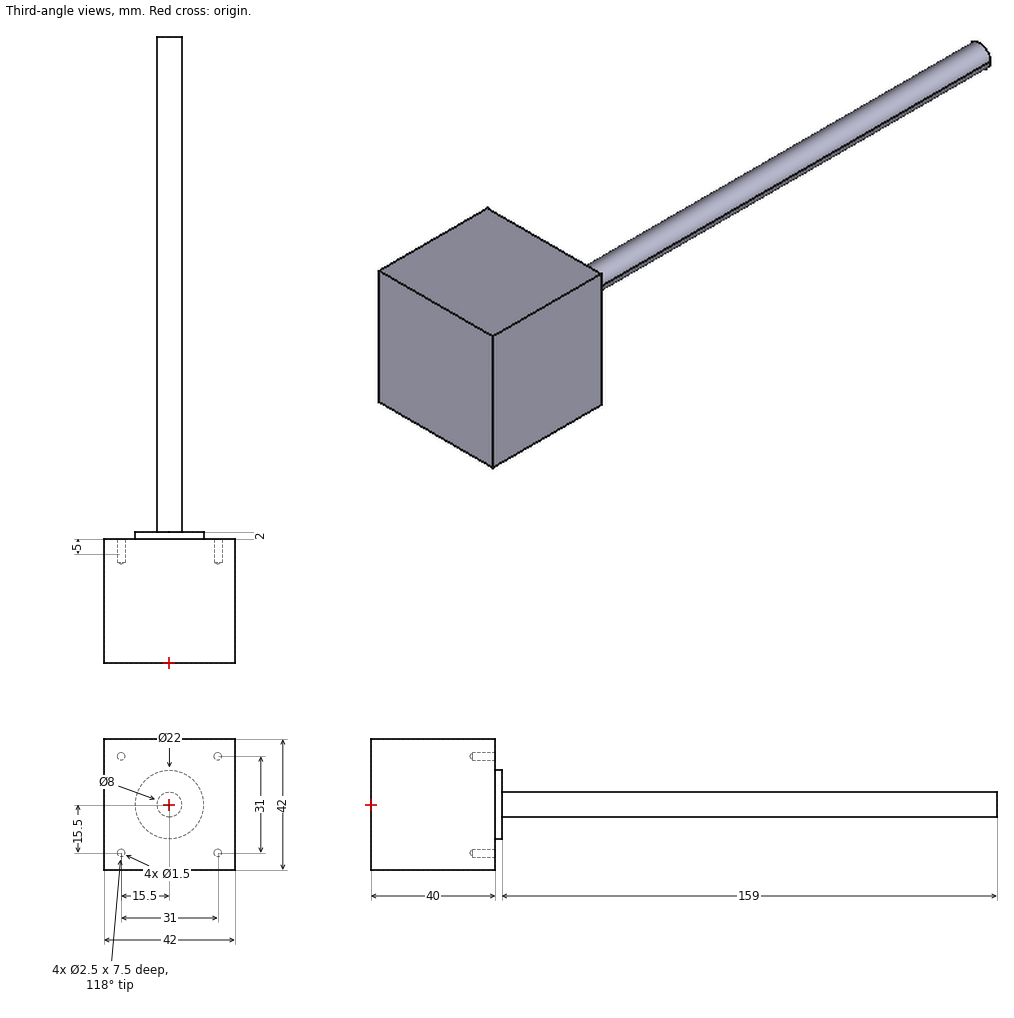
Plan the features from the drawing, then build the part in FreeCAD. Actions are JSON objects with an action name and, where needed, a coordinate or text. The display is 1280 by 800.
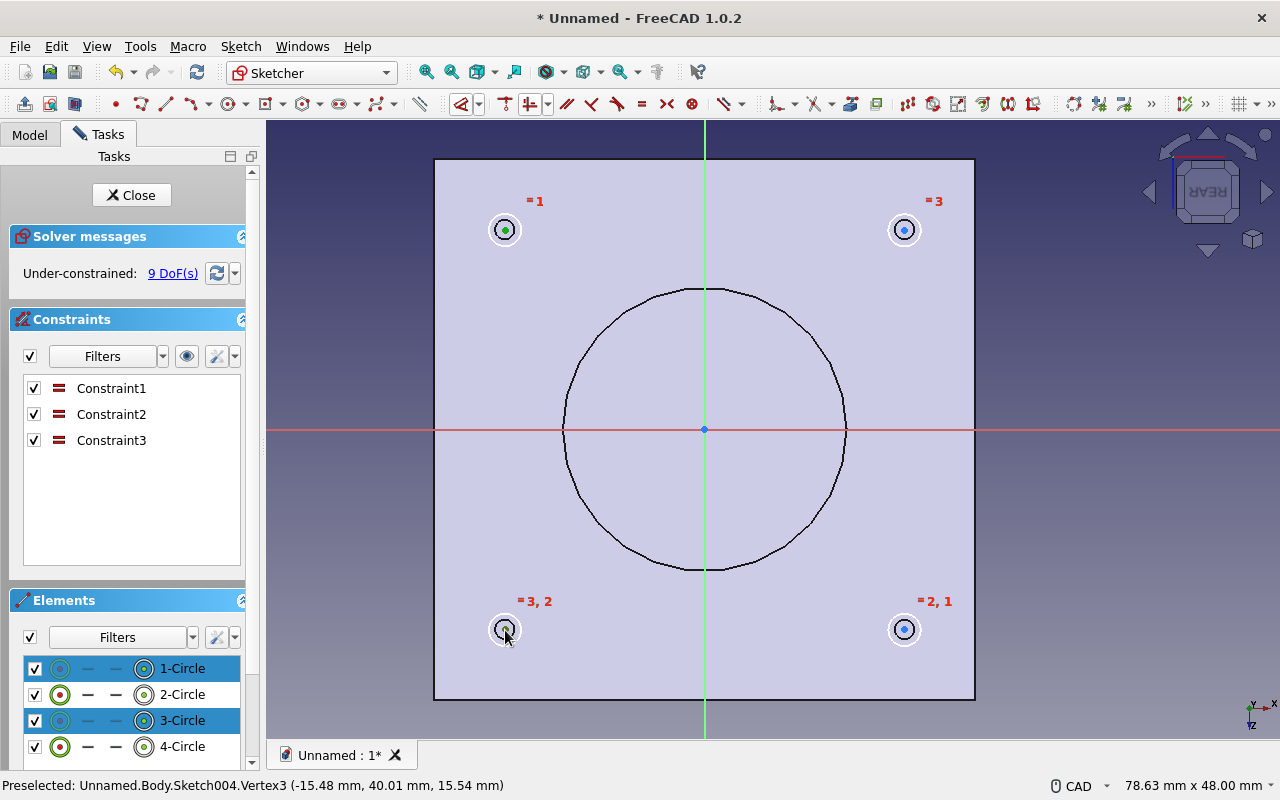
{"action": "key", "text": "v"}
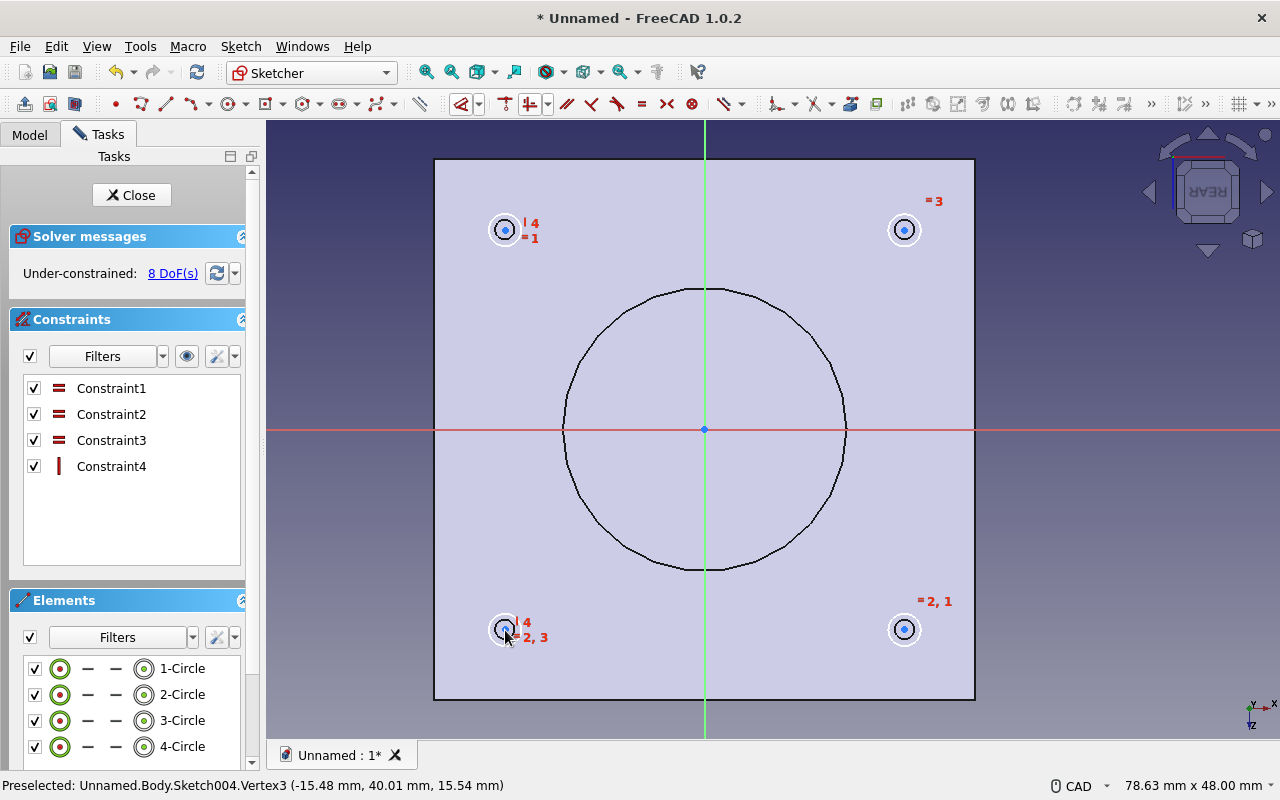
{"action": "left_click", "coordinate": [905, 630]}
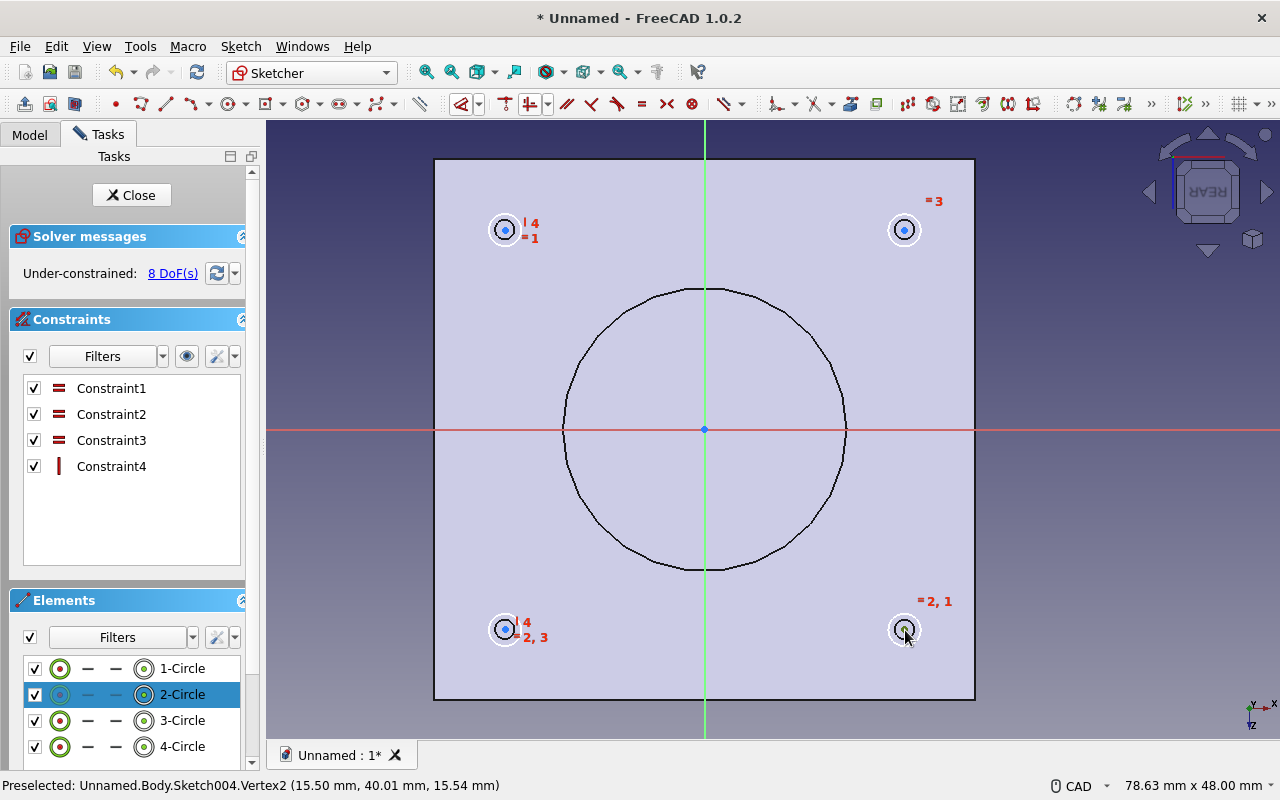
{"action": "left_click", "coordinate": [505, 630]}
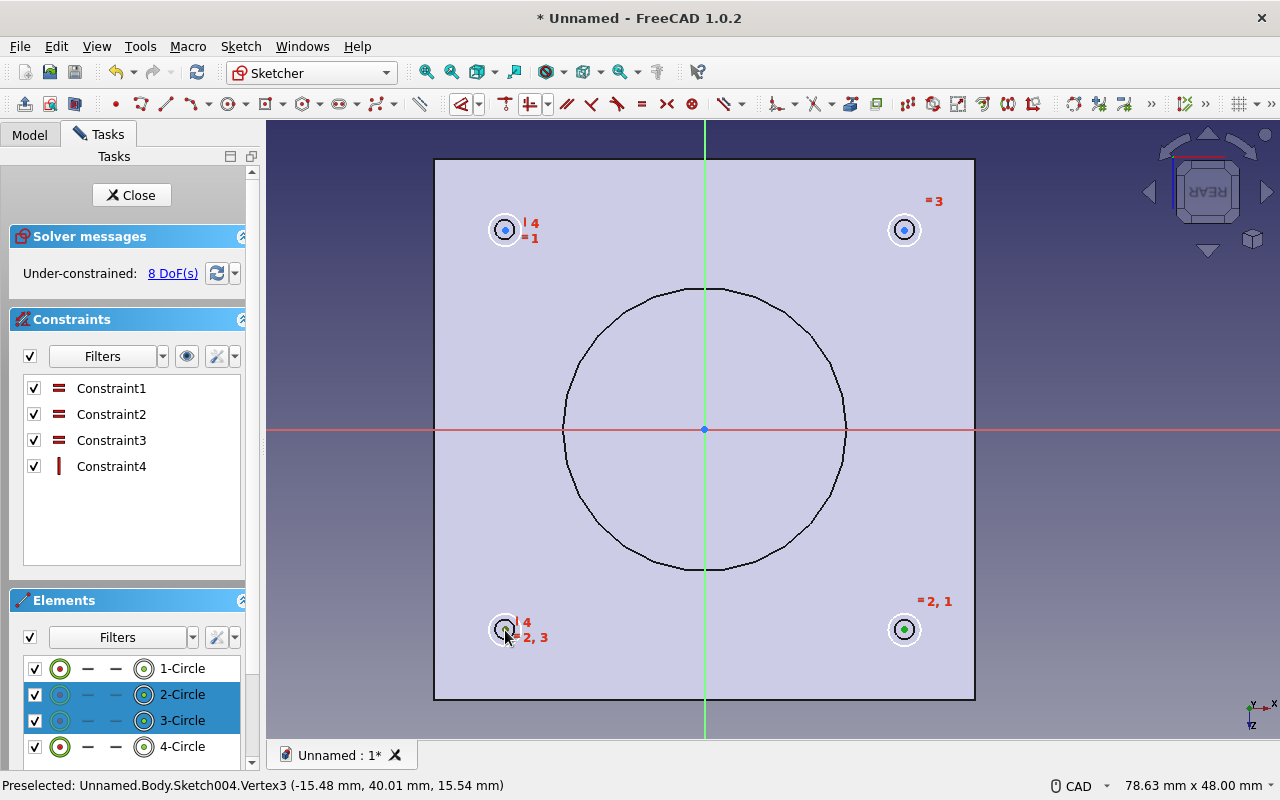
{"action": "key", "text": "h"}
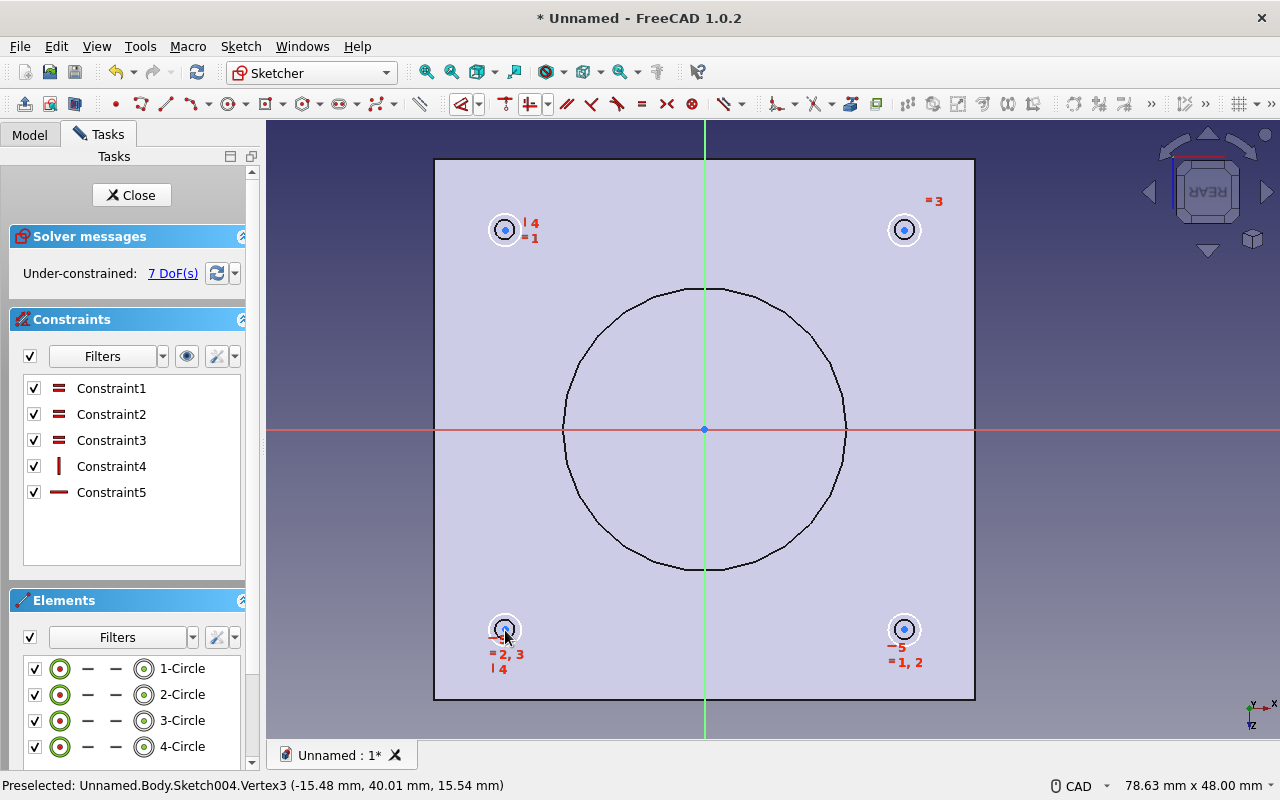
{"action": "left_click", "coordinate": [905, 630]}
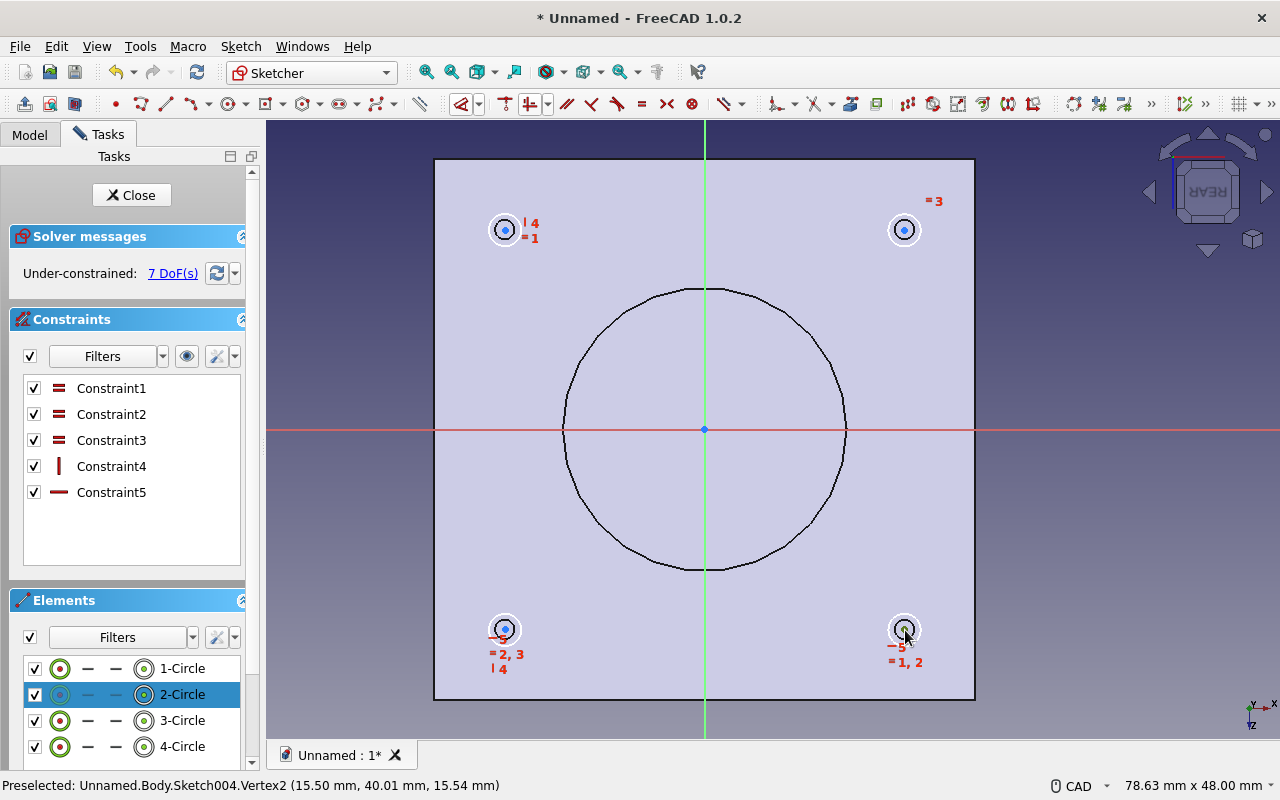
{"action": "left_click", "coordinate": [905, 230]}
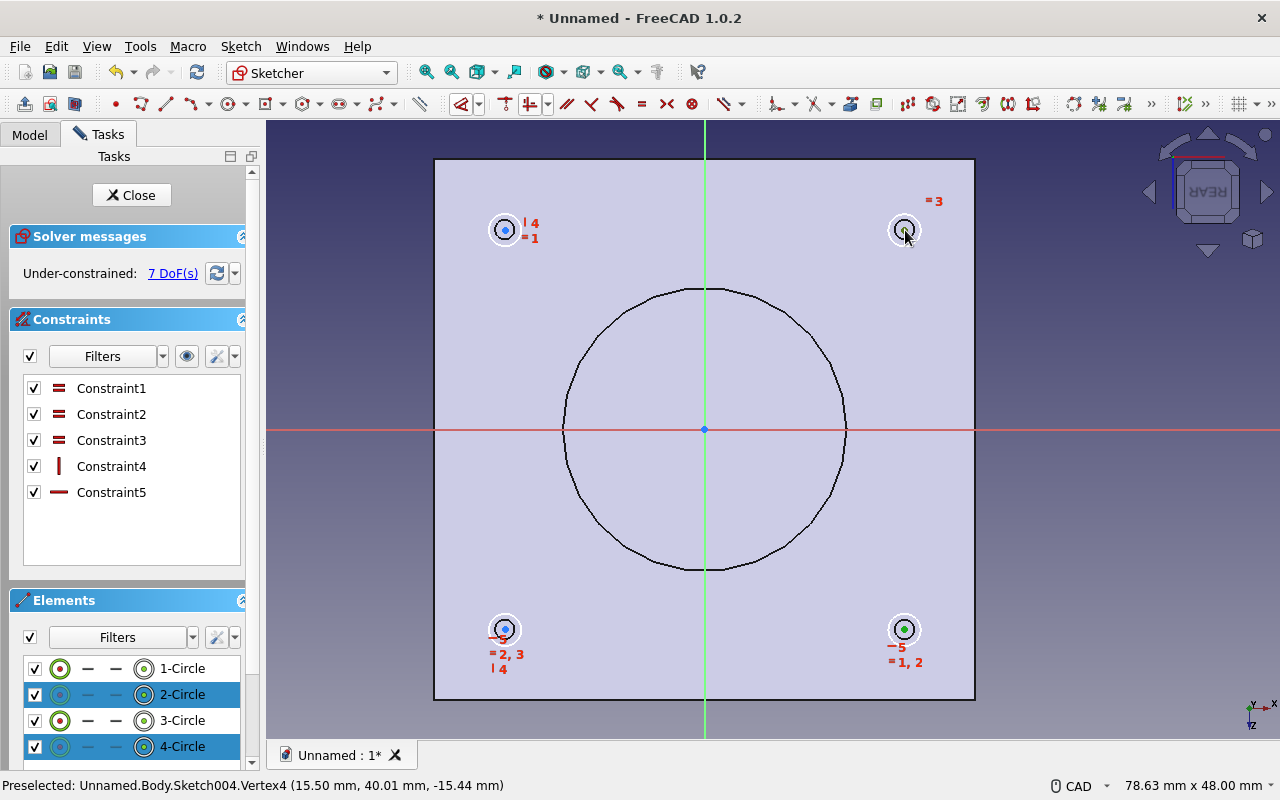
{"action": "key", "text": "v"}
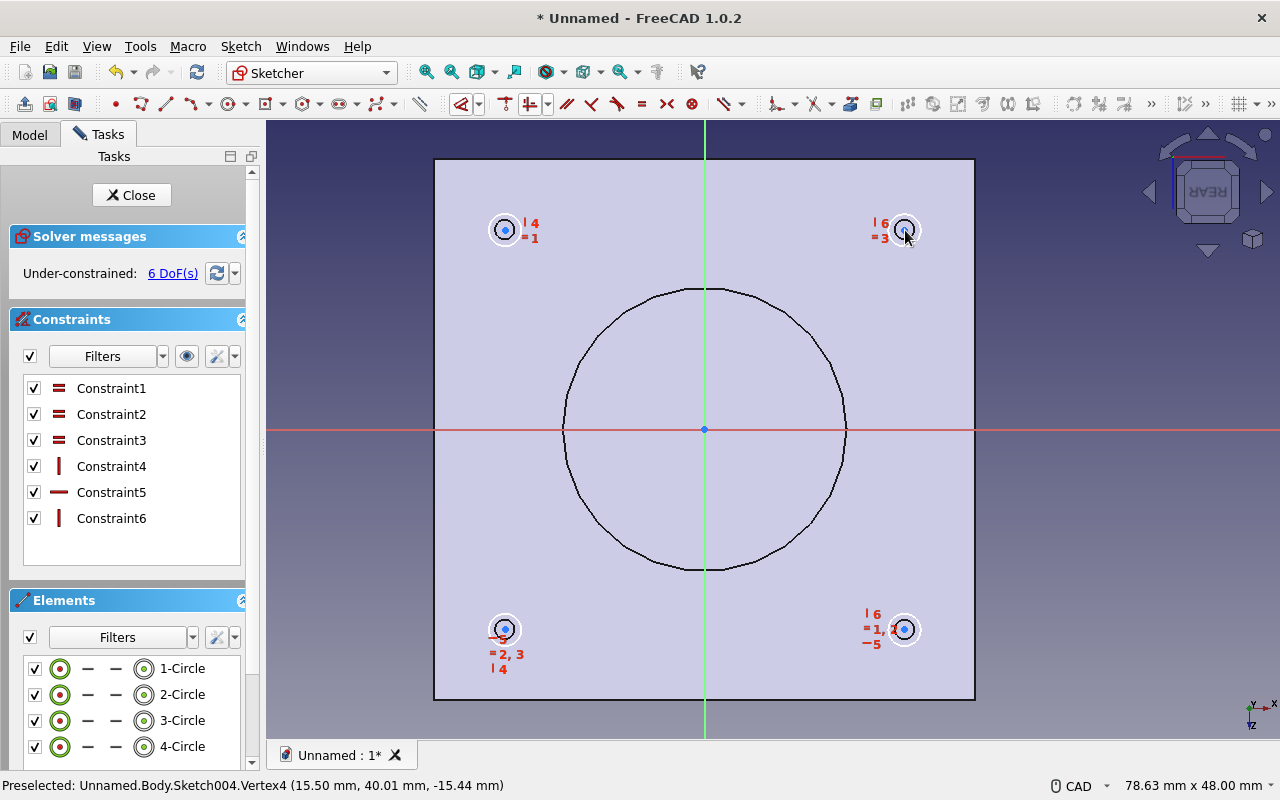
{"action": "left_click", "coordinate": [505, 230]}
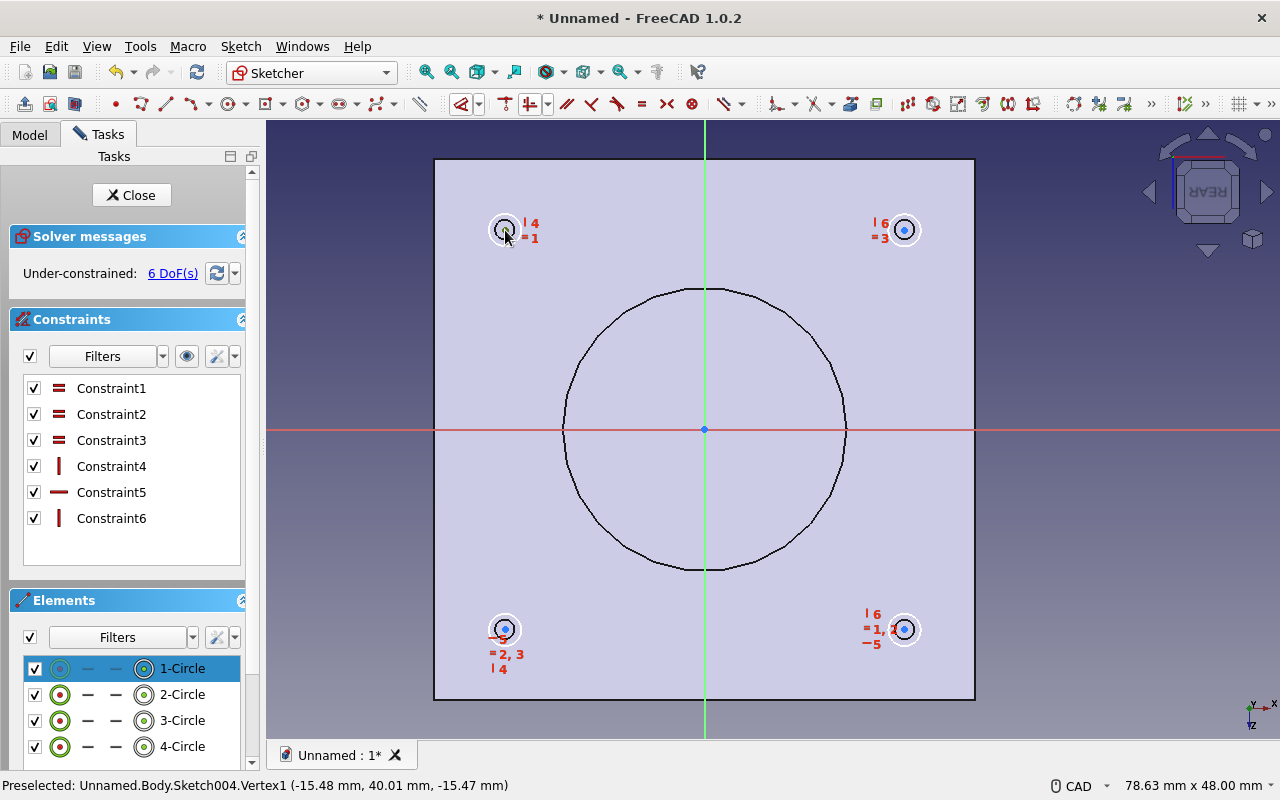
{"action": "left_click", "coordinate": [905, 230]}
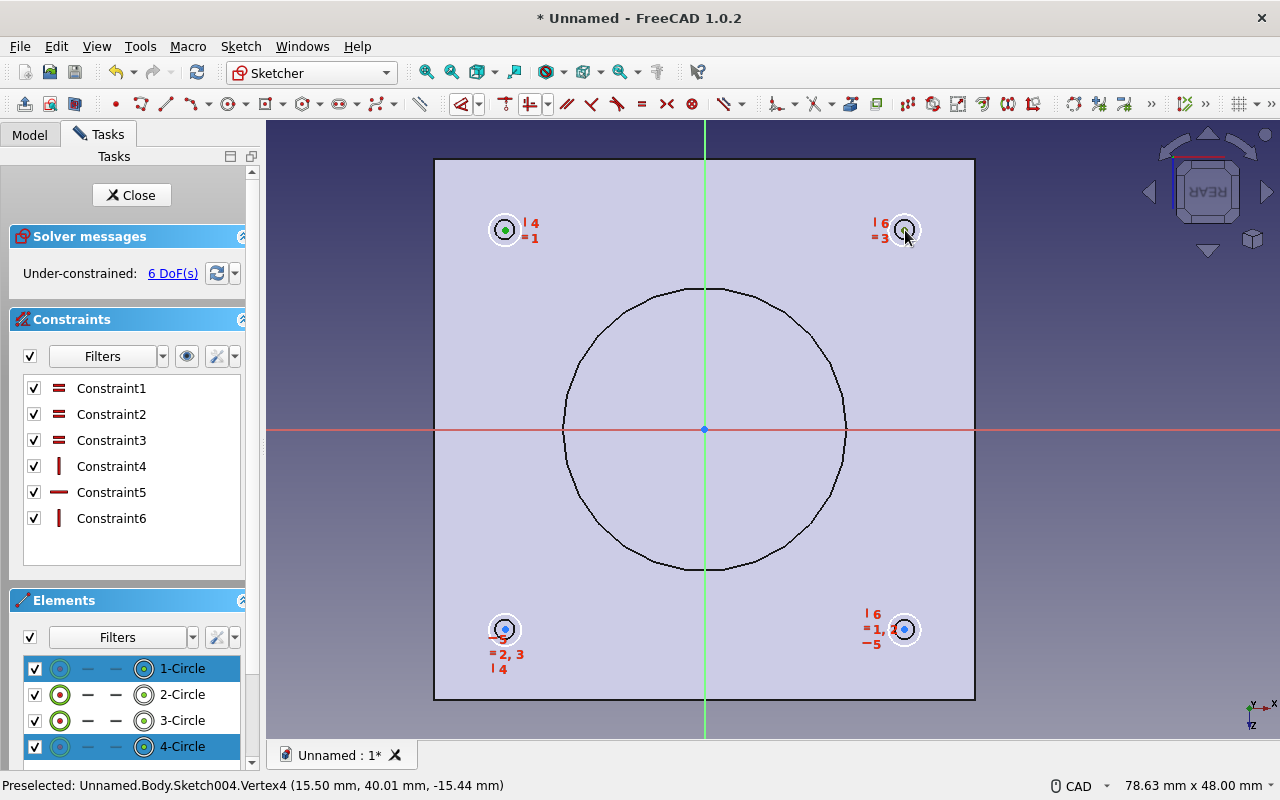
{"action": "key", "text": "h"}